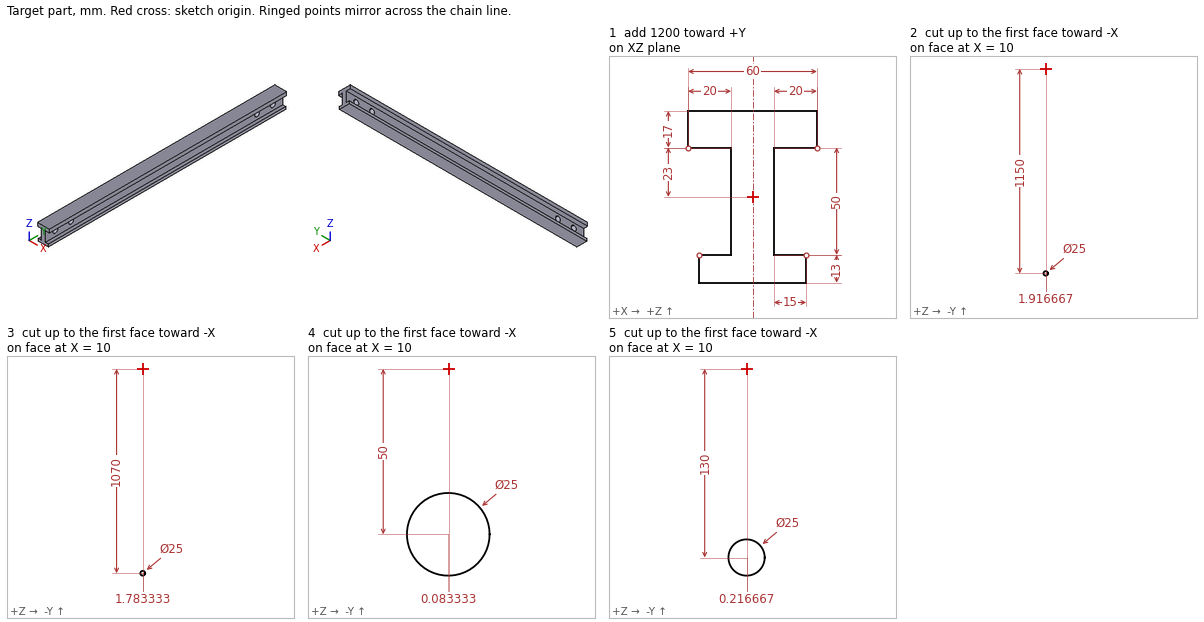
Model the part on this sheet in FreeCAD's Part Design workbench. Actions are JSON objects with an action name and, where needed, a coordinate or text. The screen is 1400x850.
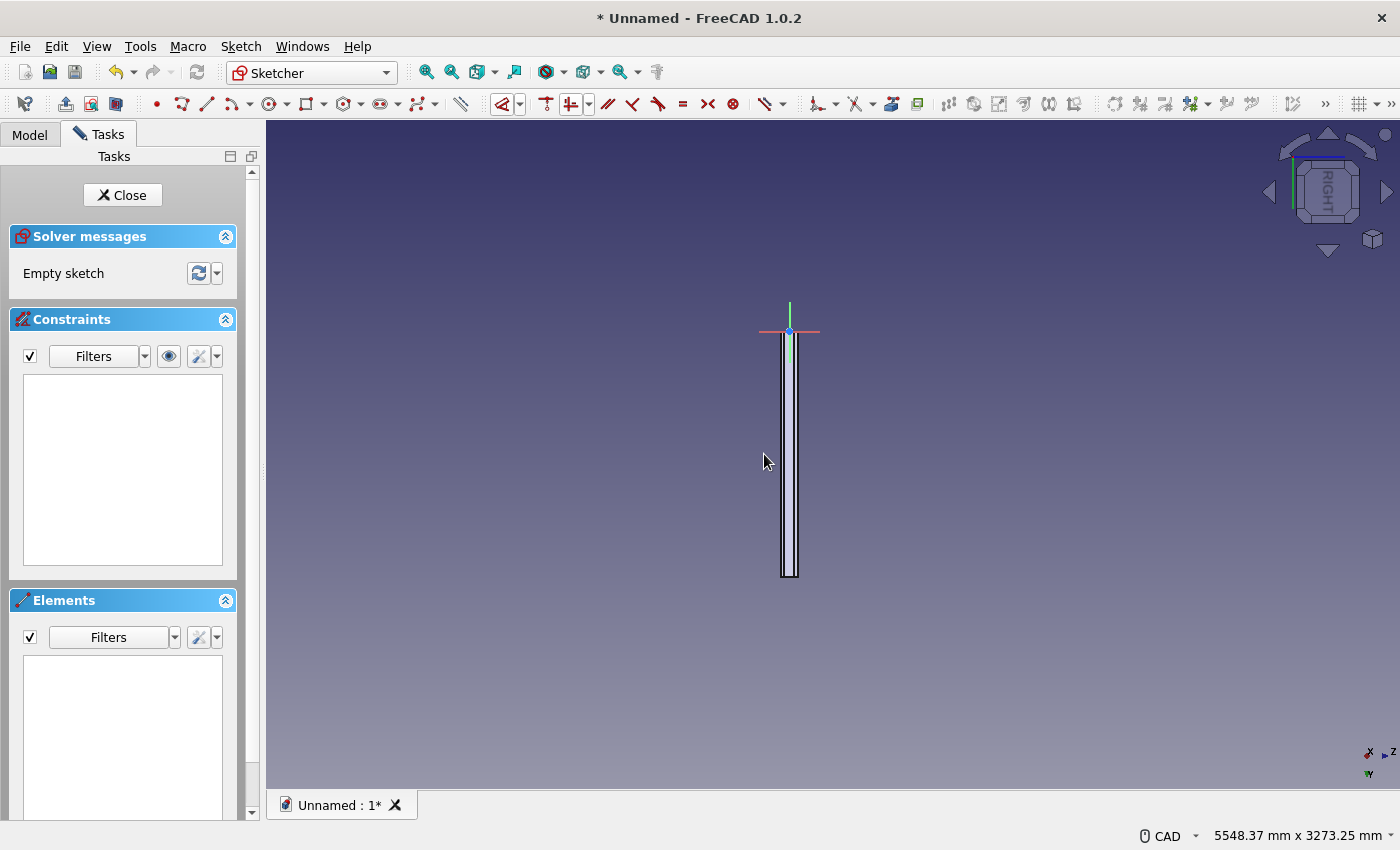
{"action": "scroll", "coordinate": [791, 573], "scroll_direction": "up", "scroll_amount": 15}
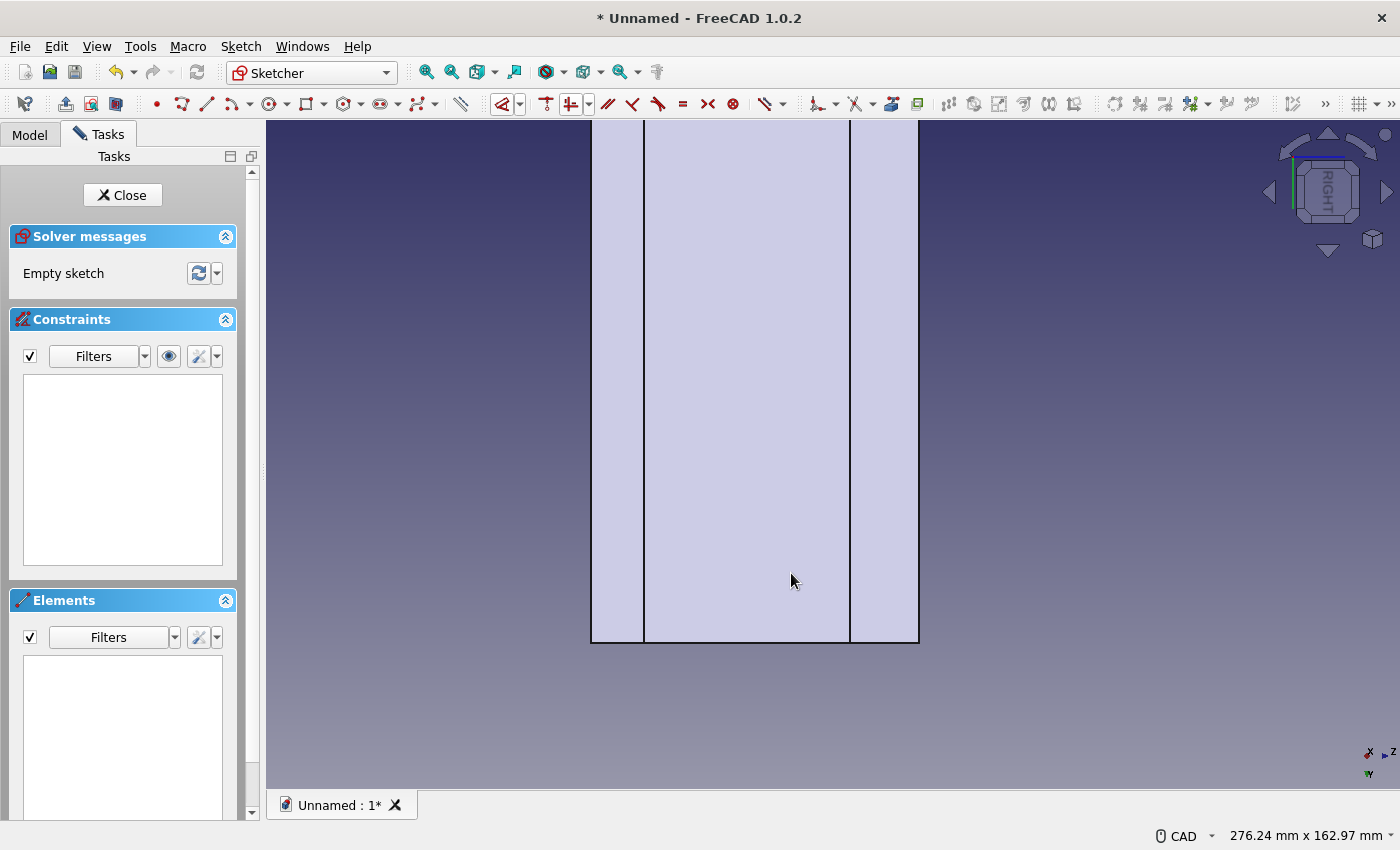
{"action": "scroll", "coordinate": [742, 432], "scroll_direction": "up", "scroll_amount": 7}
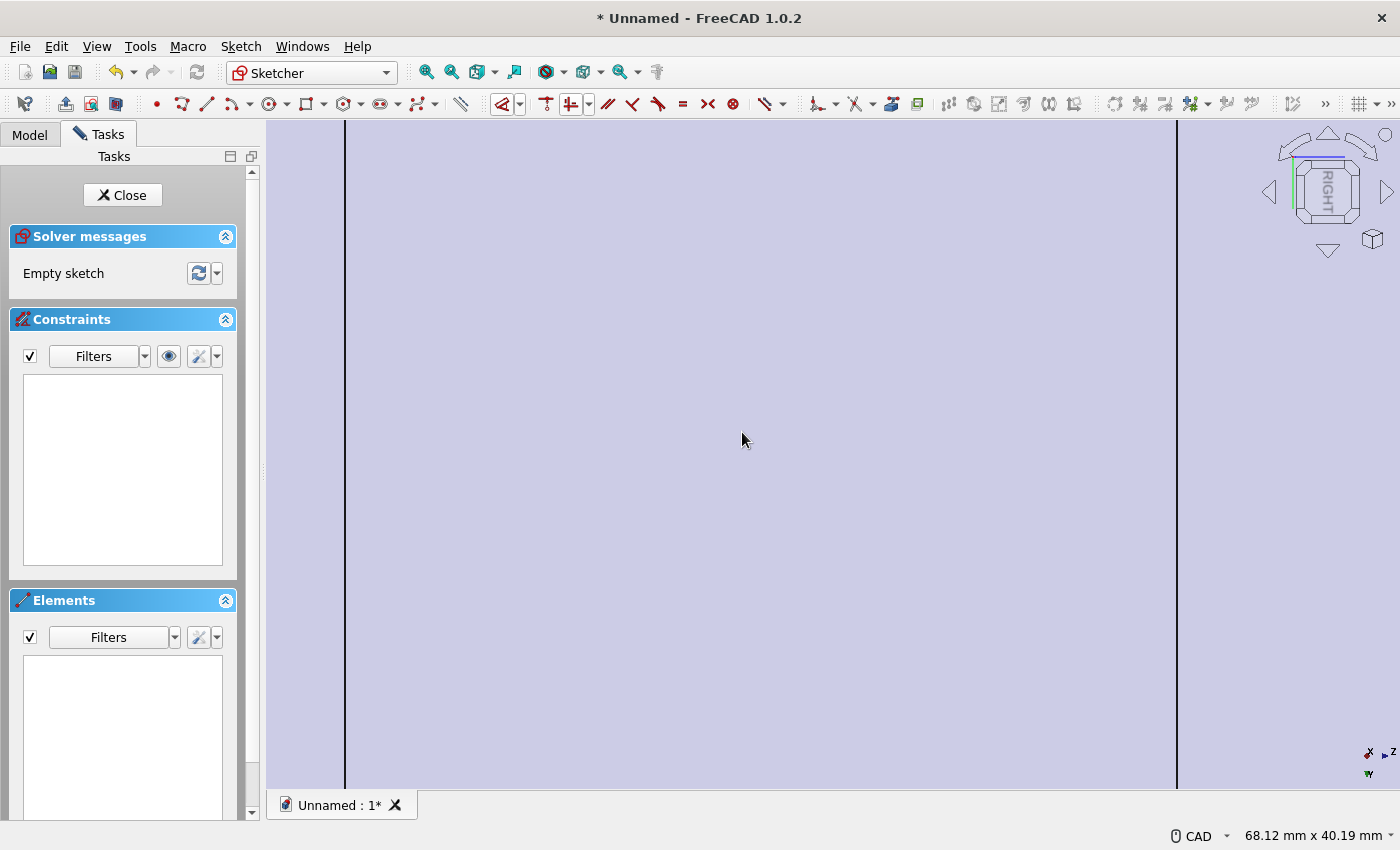
{"action": "left_click", "coordinate": [268, 104]}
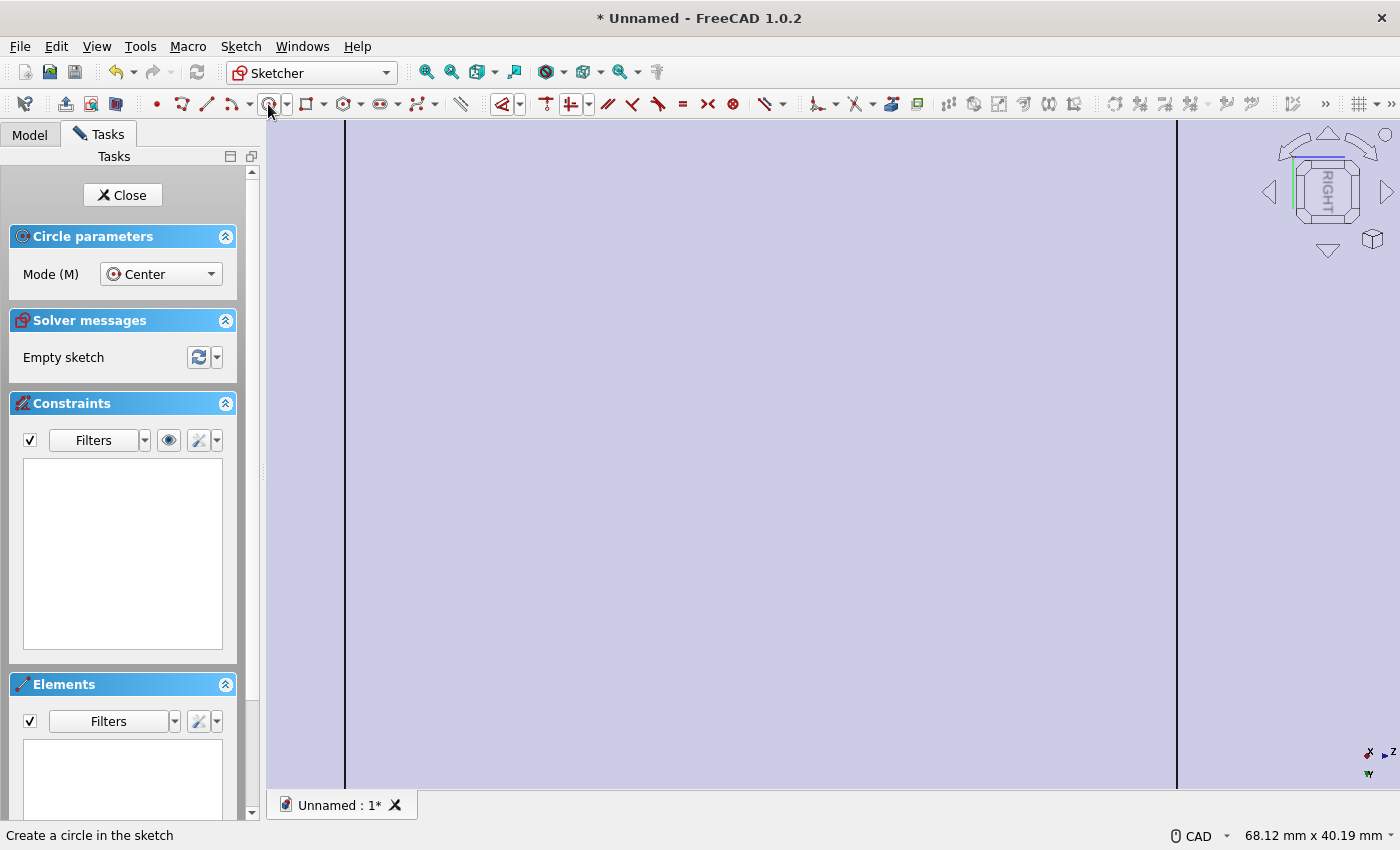
{"action": "left_click", "coordinate": [763, 454]}
{"action": "left_click", "coordinate": [910, 307]}
{"action": "key", "text": "Escape"}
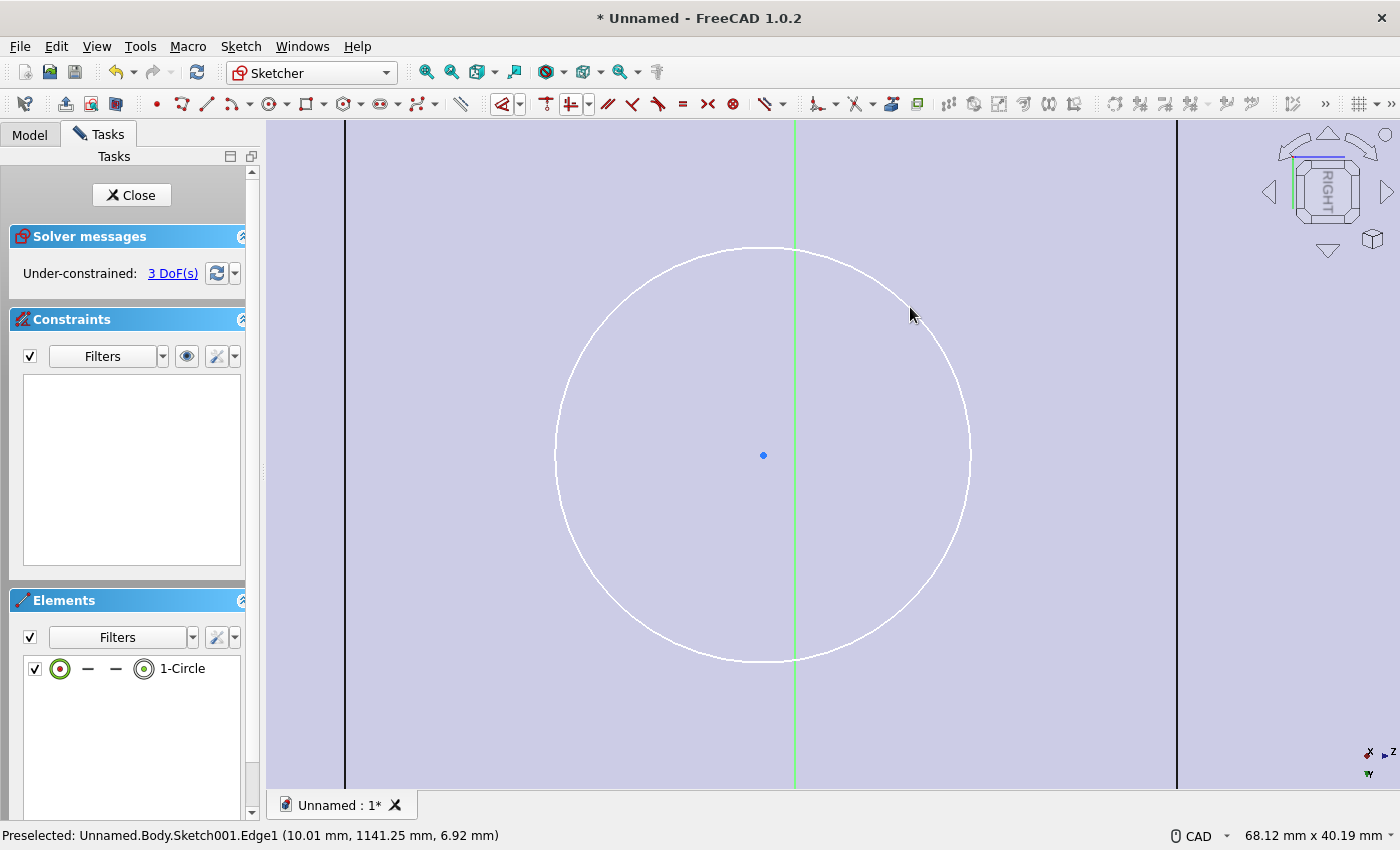
{"action": "left_click", "coordinate": [910, 308]}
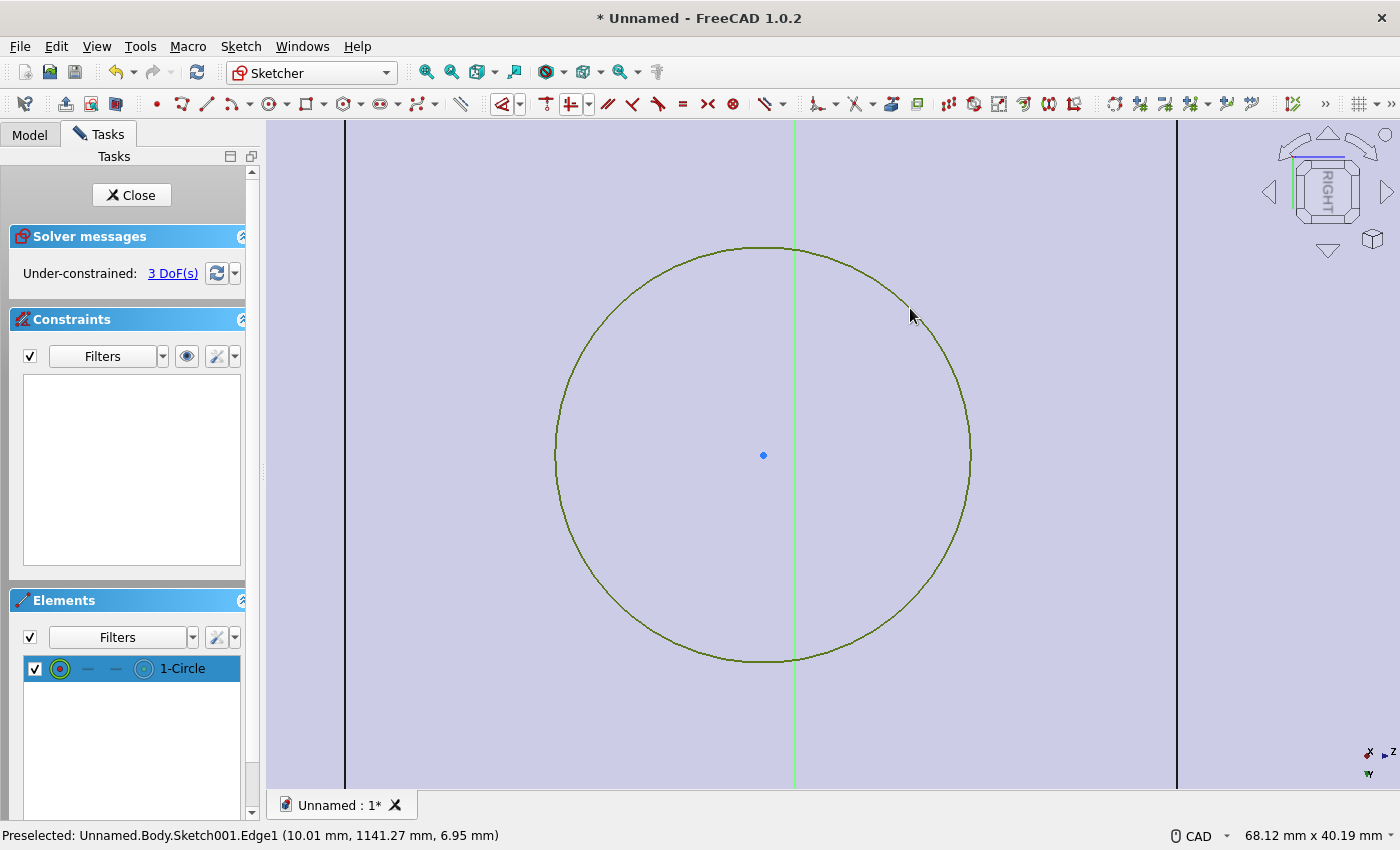
{"action": "key", "text": "k o"}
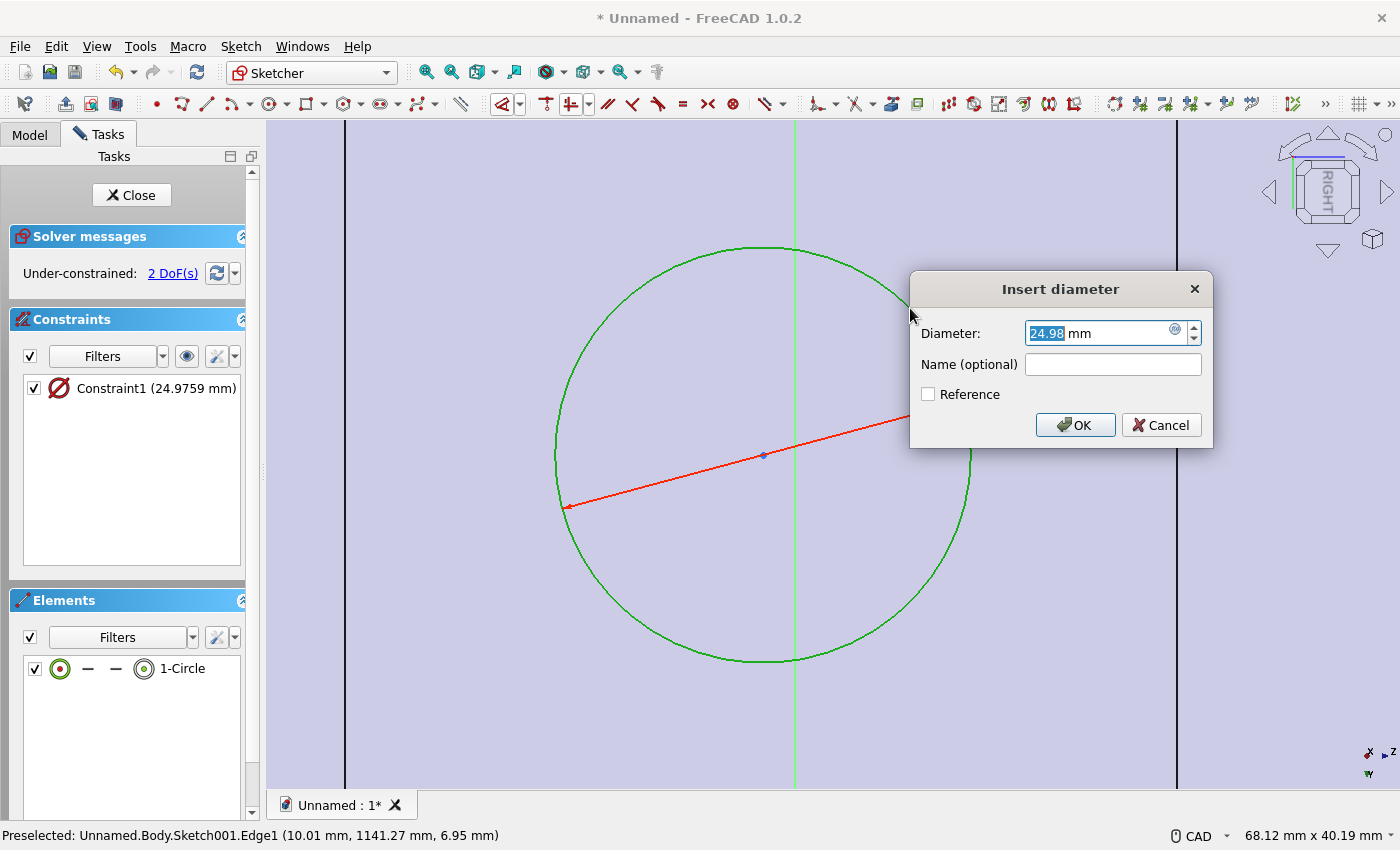
{"action": "type", "text": "25"}
{"action": "key", "text": "Return"}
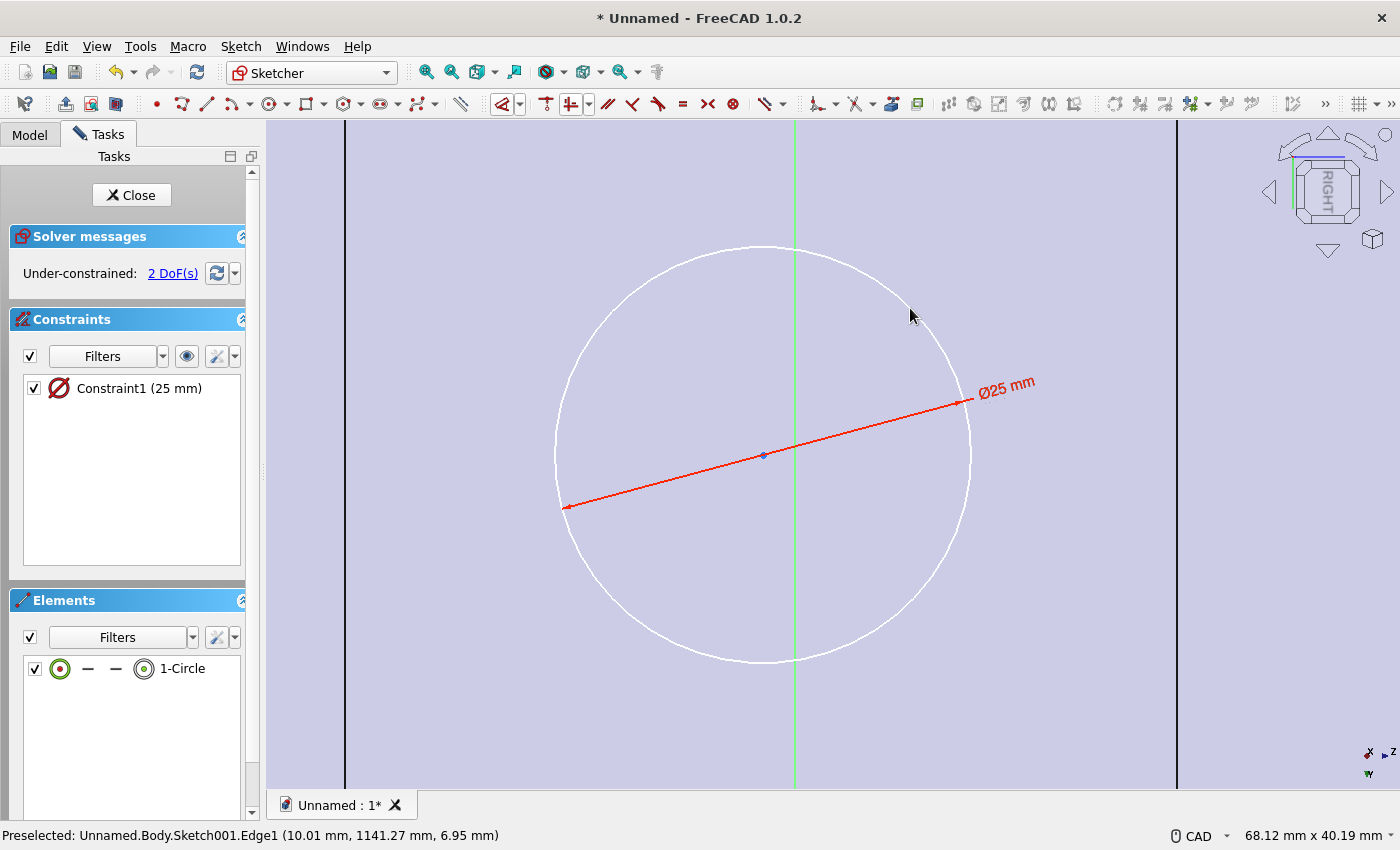
{"action": "left_click", "coordinate": [763, 455]}